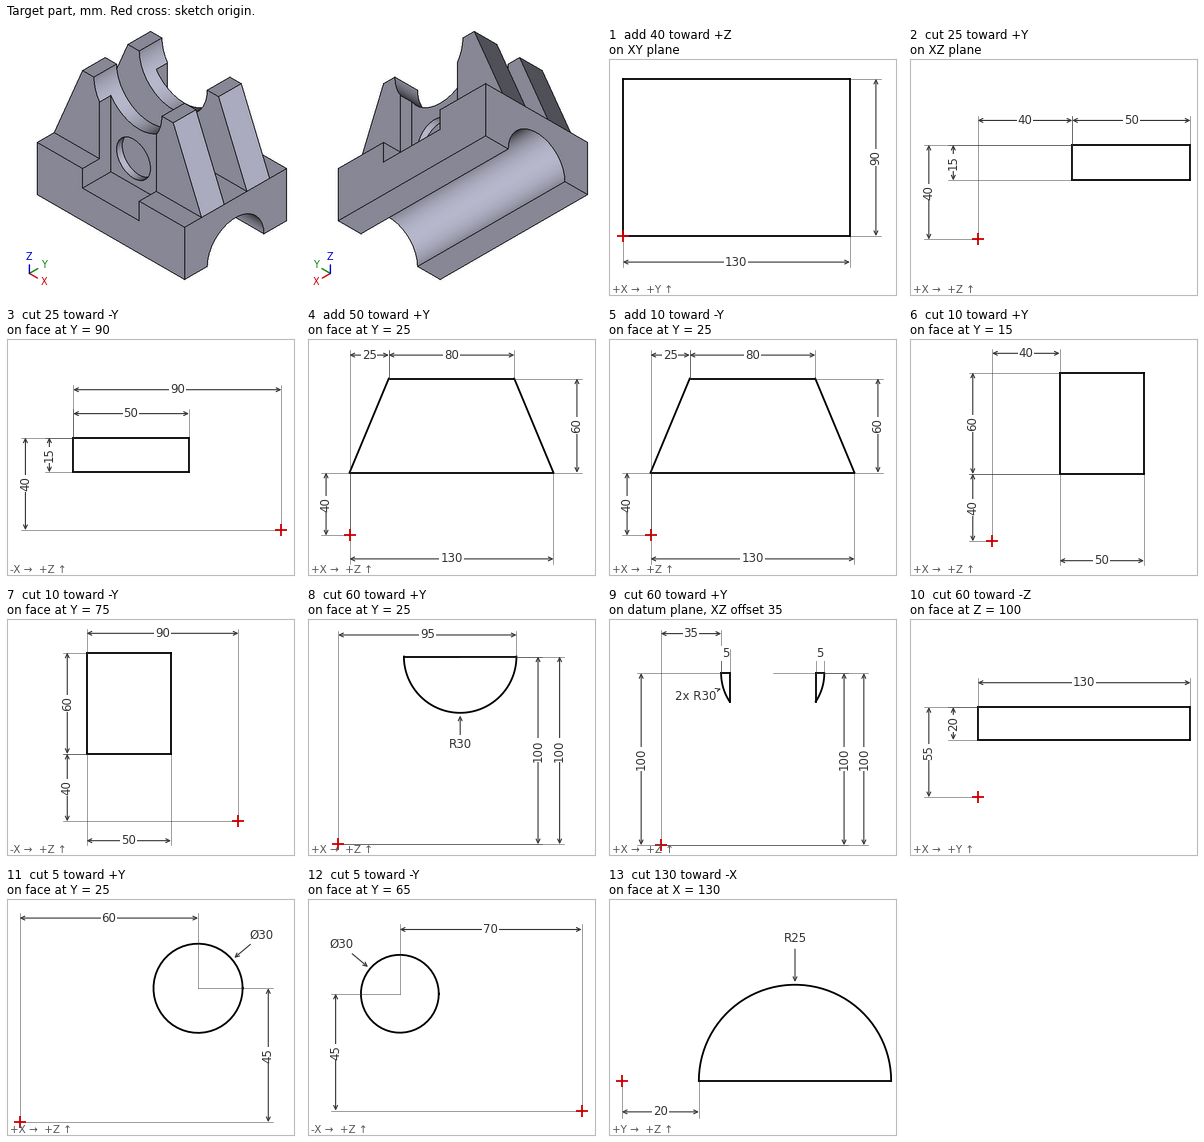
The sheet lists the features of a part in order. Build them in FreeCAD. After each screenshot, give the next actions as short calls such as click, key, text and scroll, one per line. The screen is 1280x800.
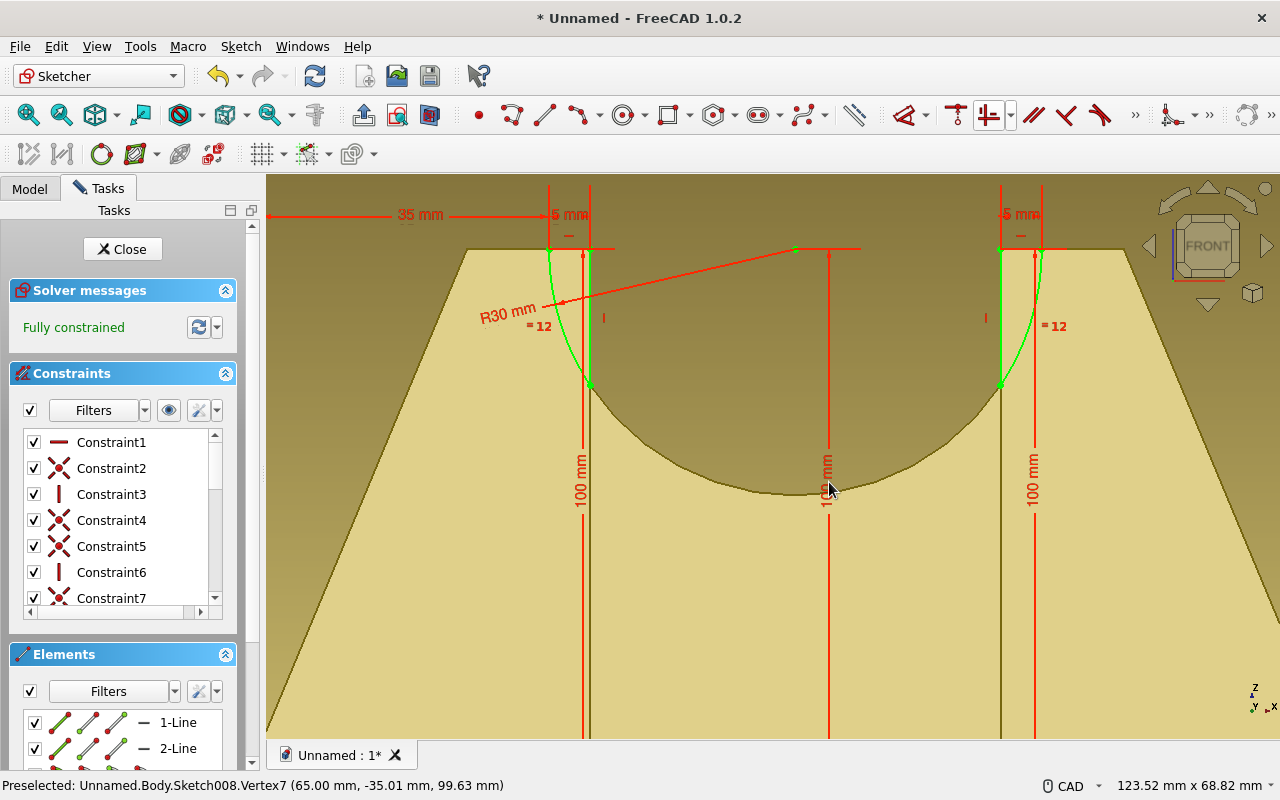
click(123, 249)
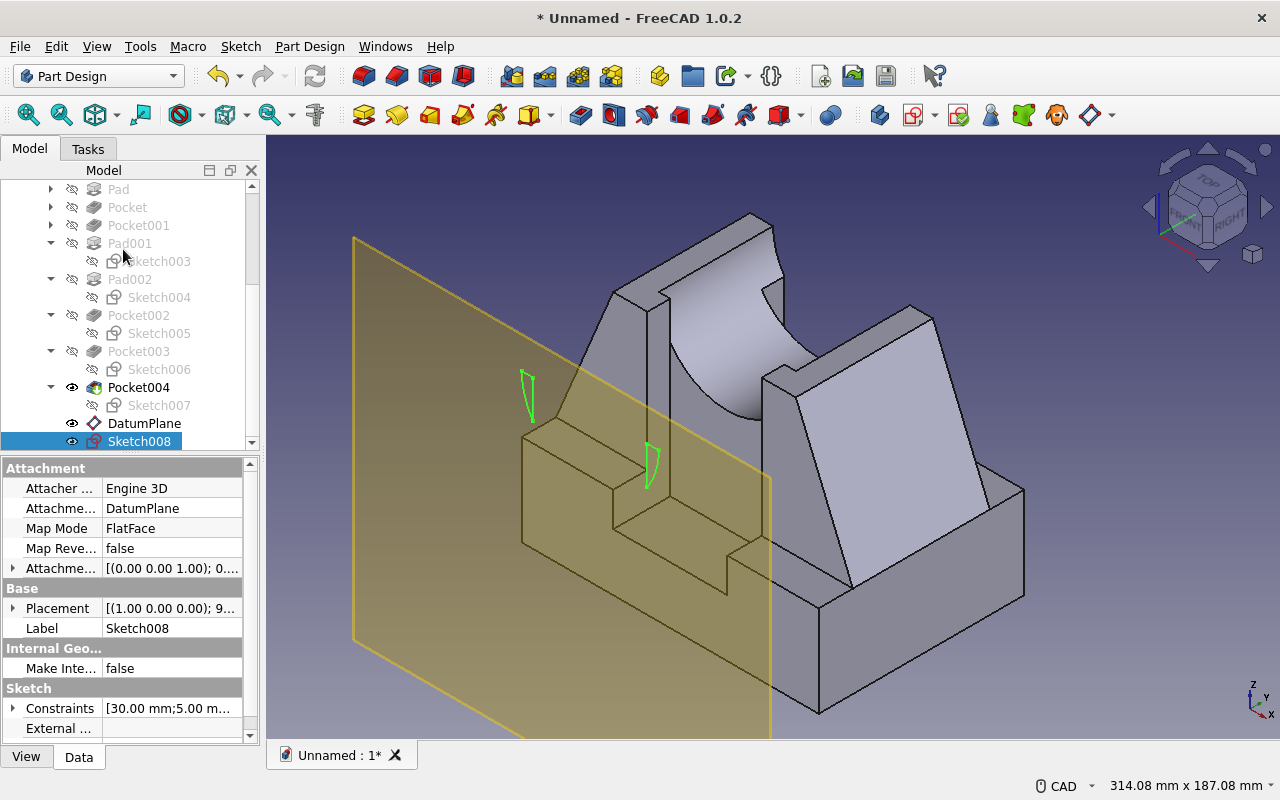
click(581, 116)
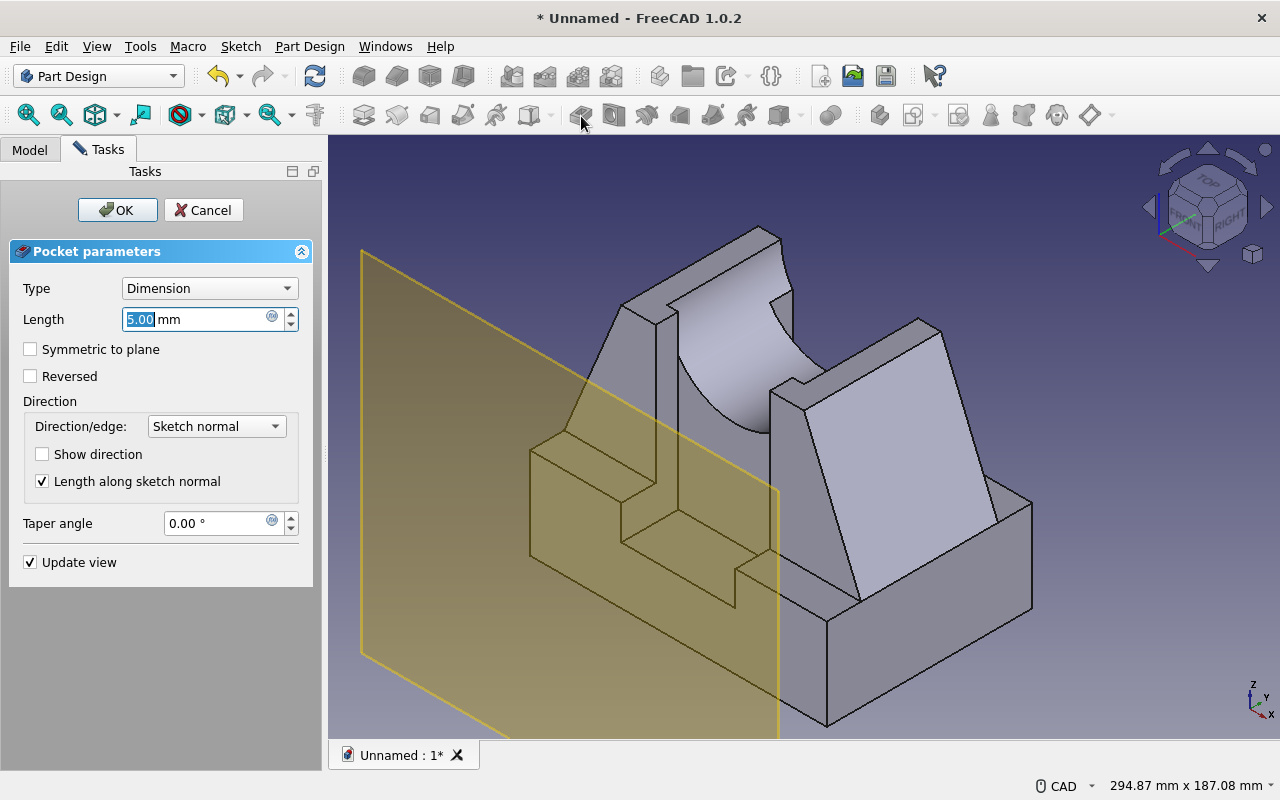
text(60)
key(Tab)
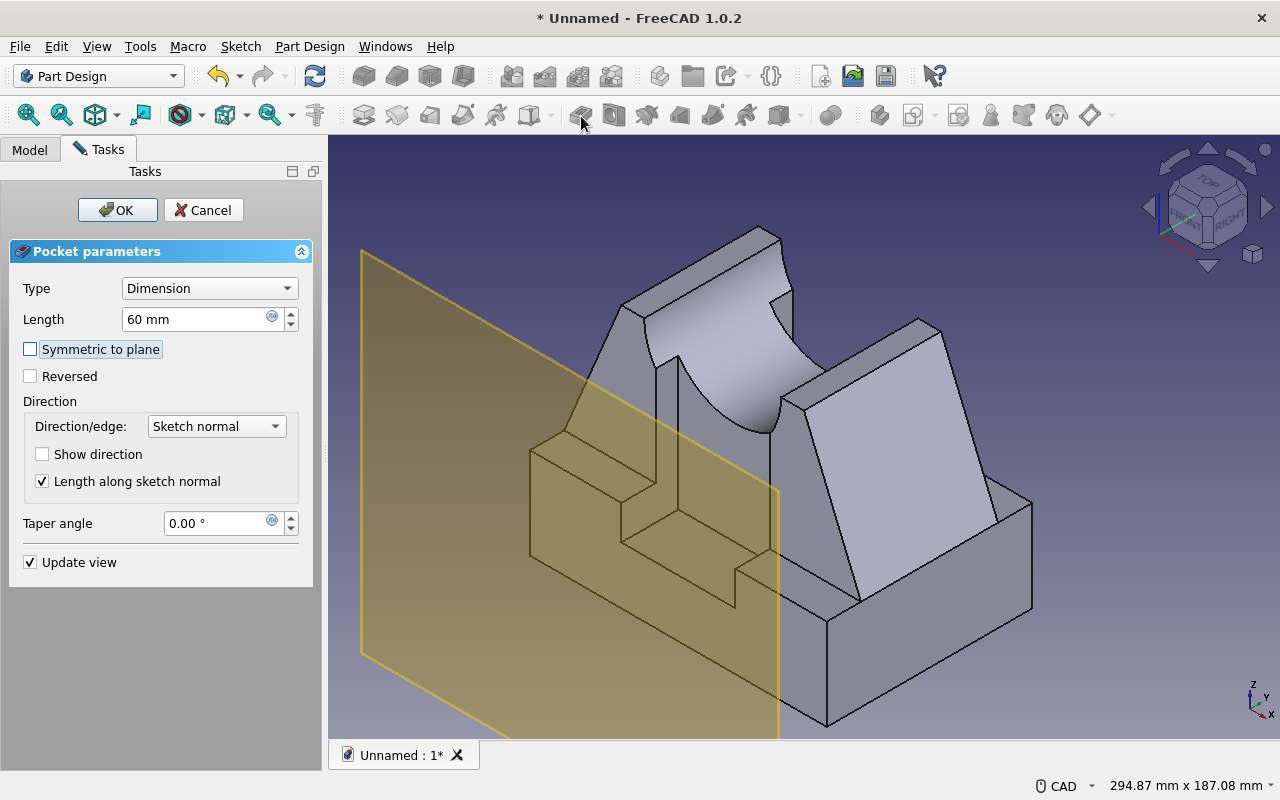
click(118, 210)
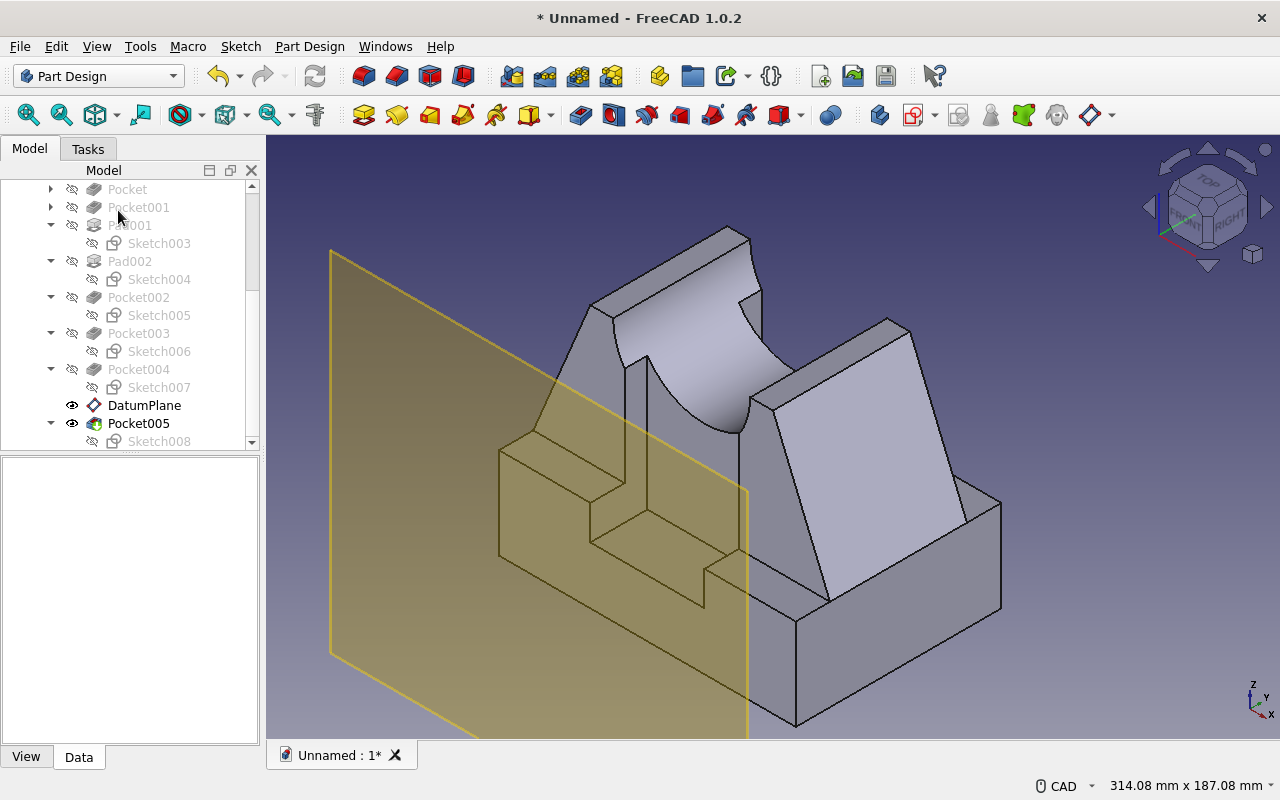
click(117, 405)
key(space)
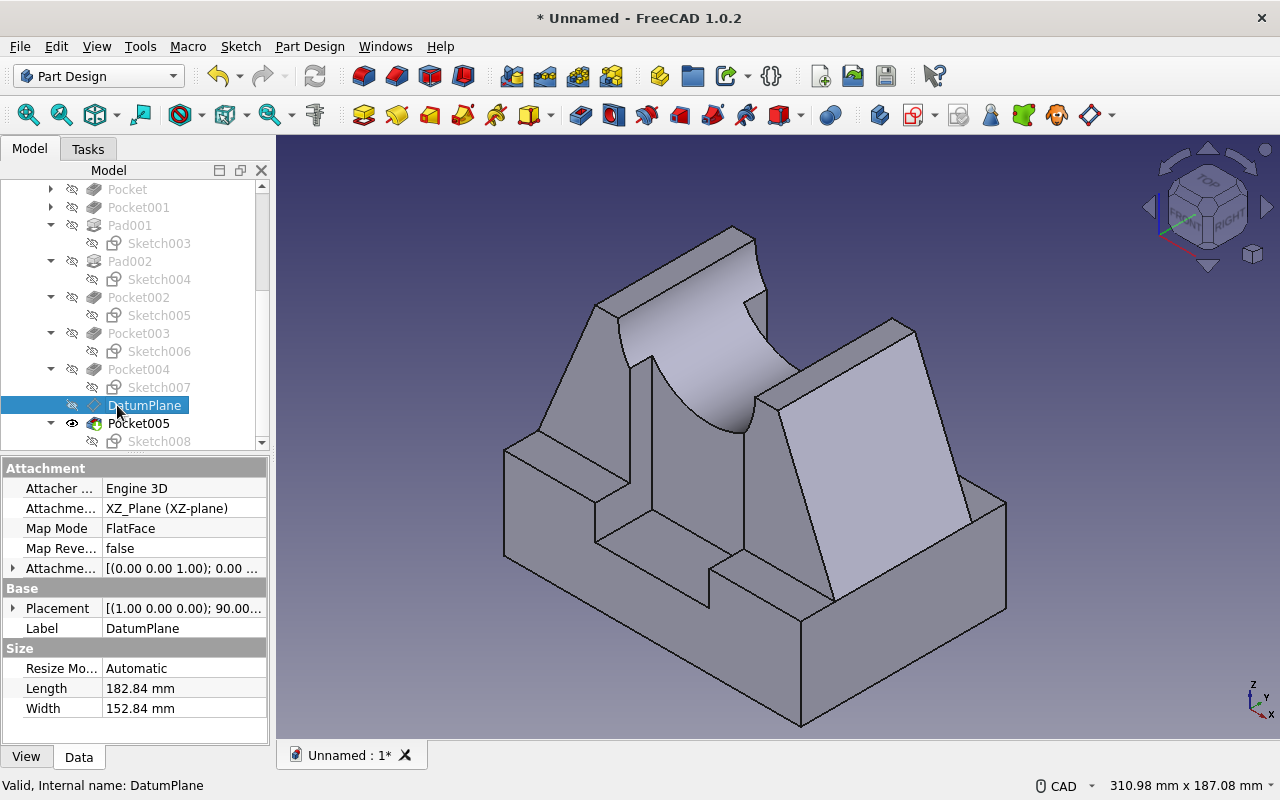
click(714, 249)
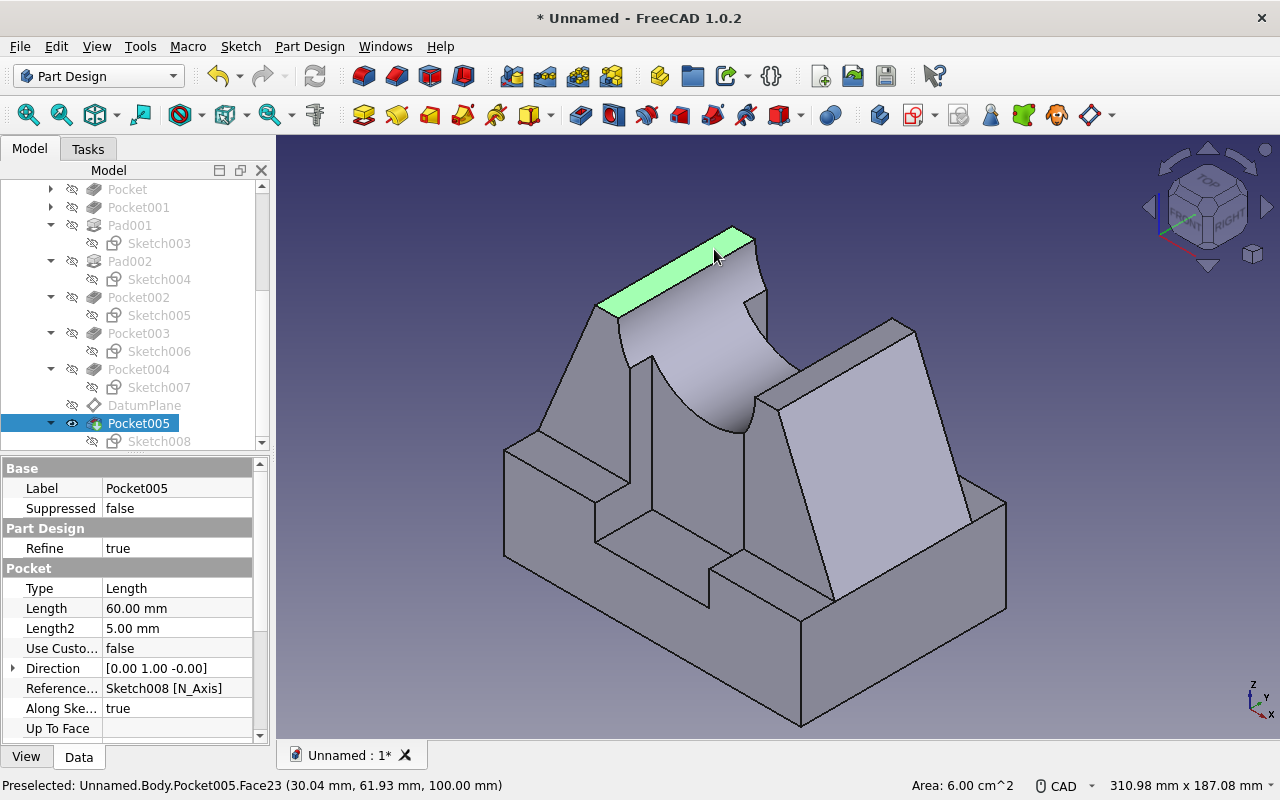
click(912, 116)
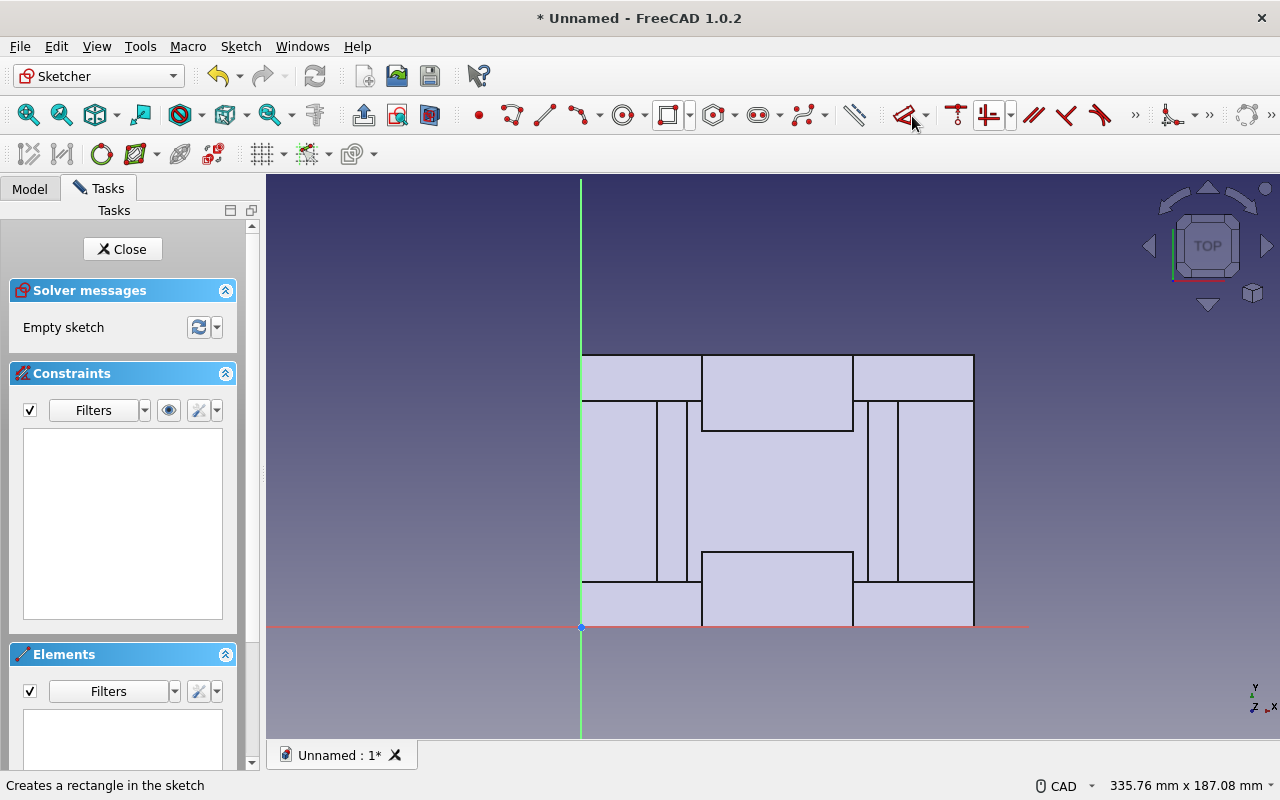
scroll(926, 711, up, 2)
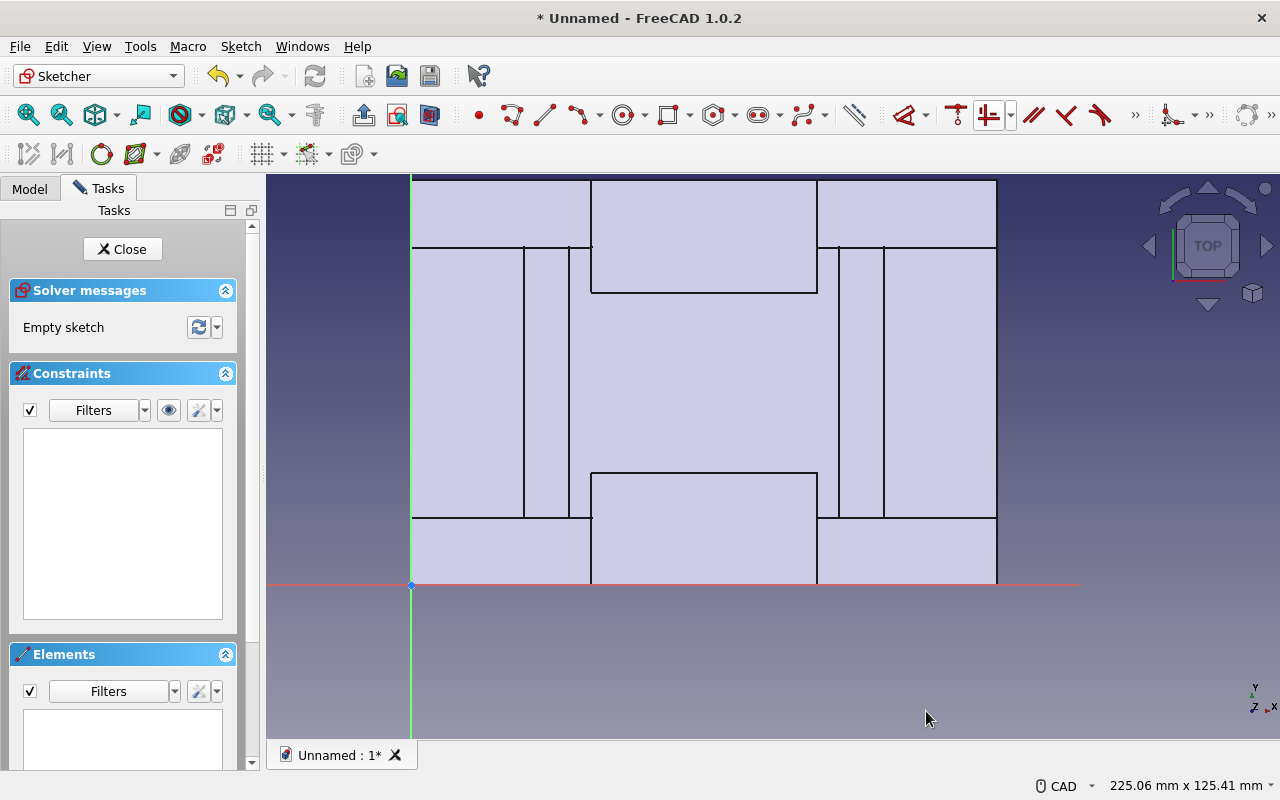
key(g)
key(r)